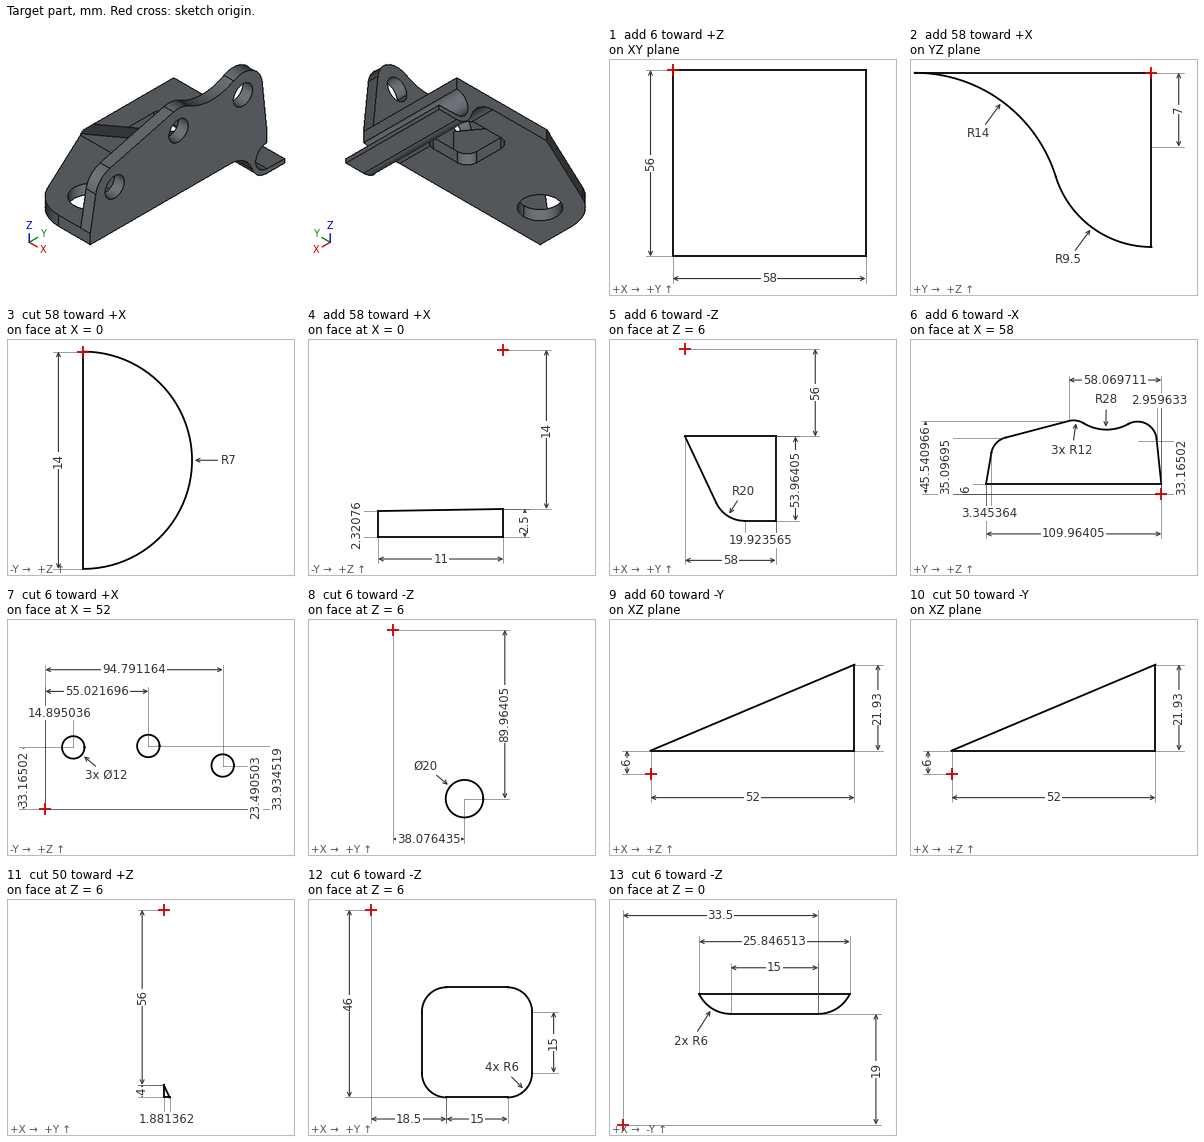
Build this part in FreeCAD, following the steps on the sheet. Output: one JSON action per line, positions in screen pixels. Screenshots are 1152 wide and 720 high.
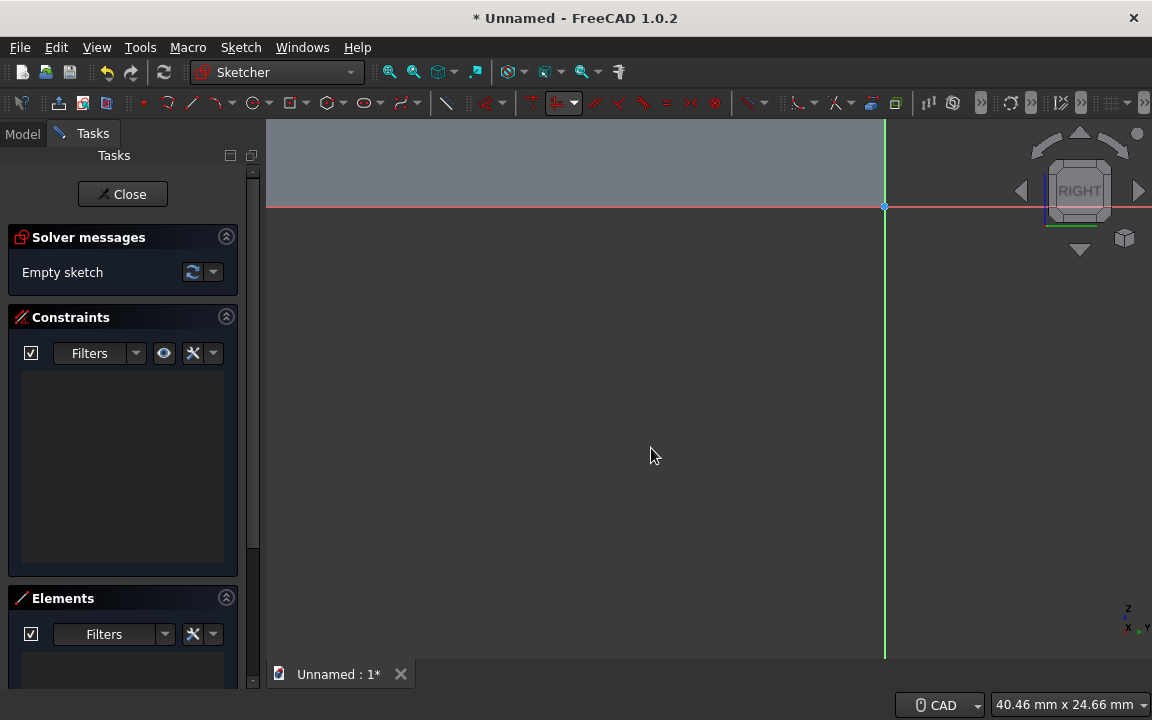
{"action": "left_click", "coordinate": [168, 104]}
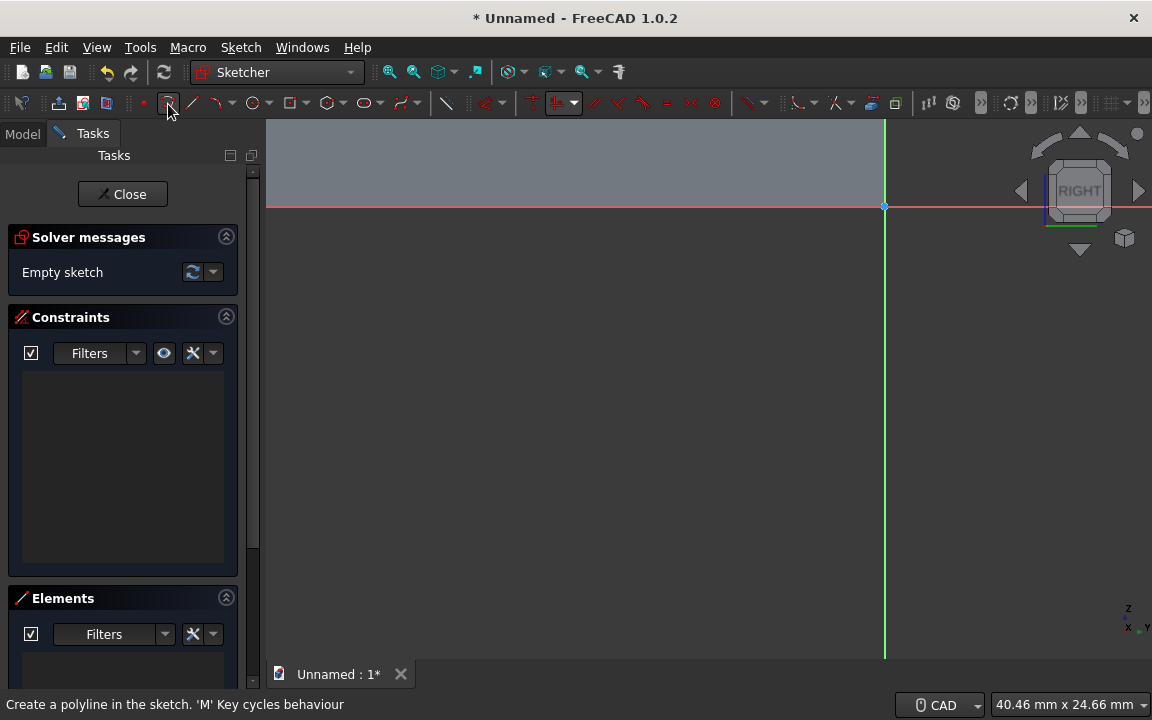
{"action": "left_click", "coordinate": [394, 207]}
{"action": "left_click", "coordinate": [885, 207]}
{"action": "left_click", "coordinate": [876, 568]}
{"action": "right_click", "coordinate": [876, 568]}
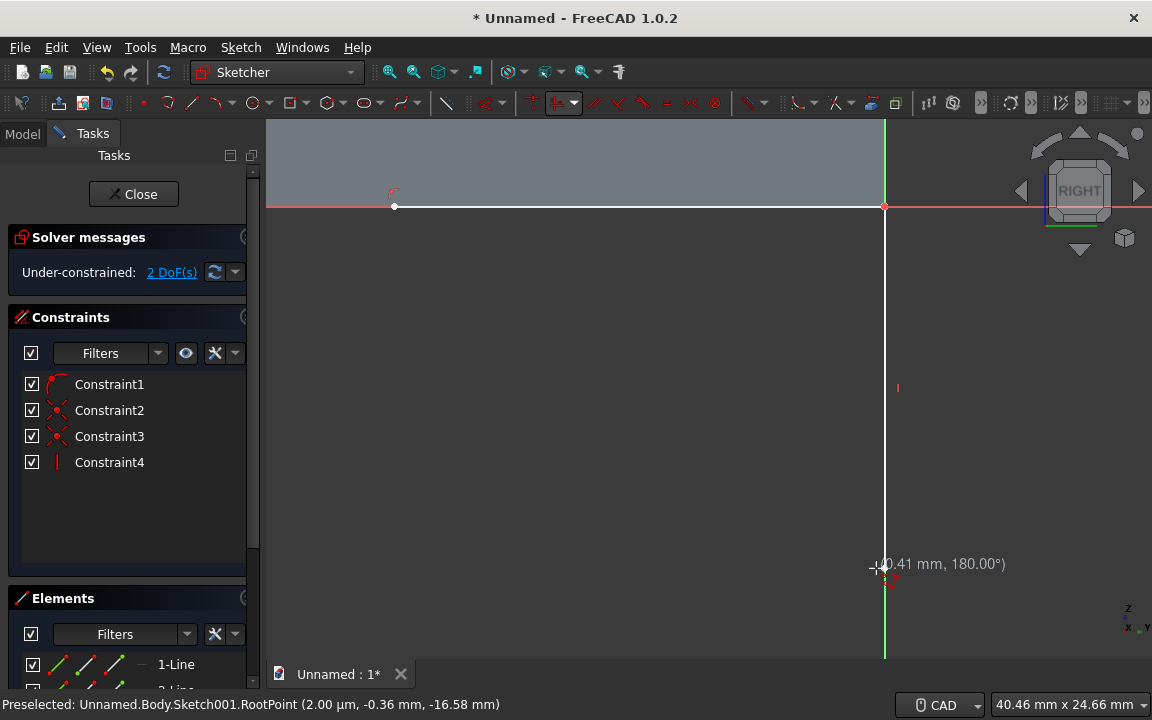
{"action": "left_click", "coordinate": [216, 104]}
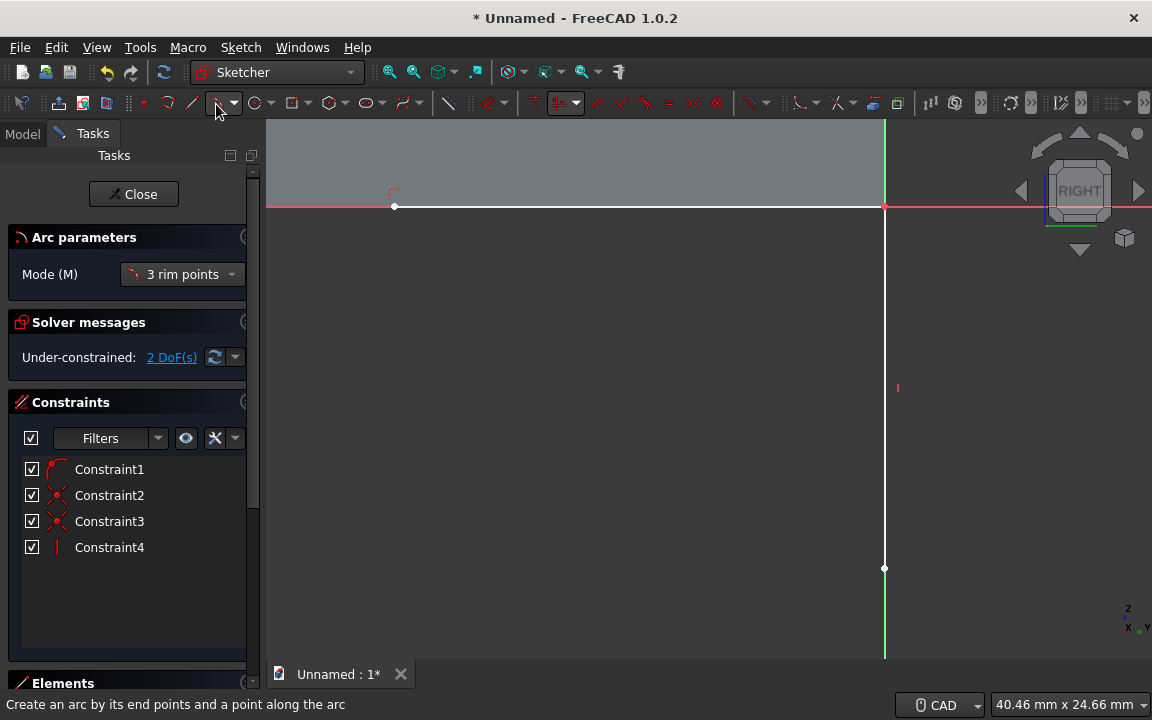
{"action": "left_click", "coordinate": [885, 569]}
{"action": "left_click", "coordinate": [686, 422]}
{"action": "left_click", "coordinate": [762, 528]}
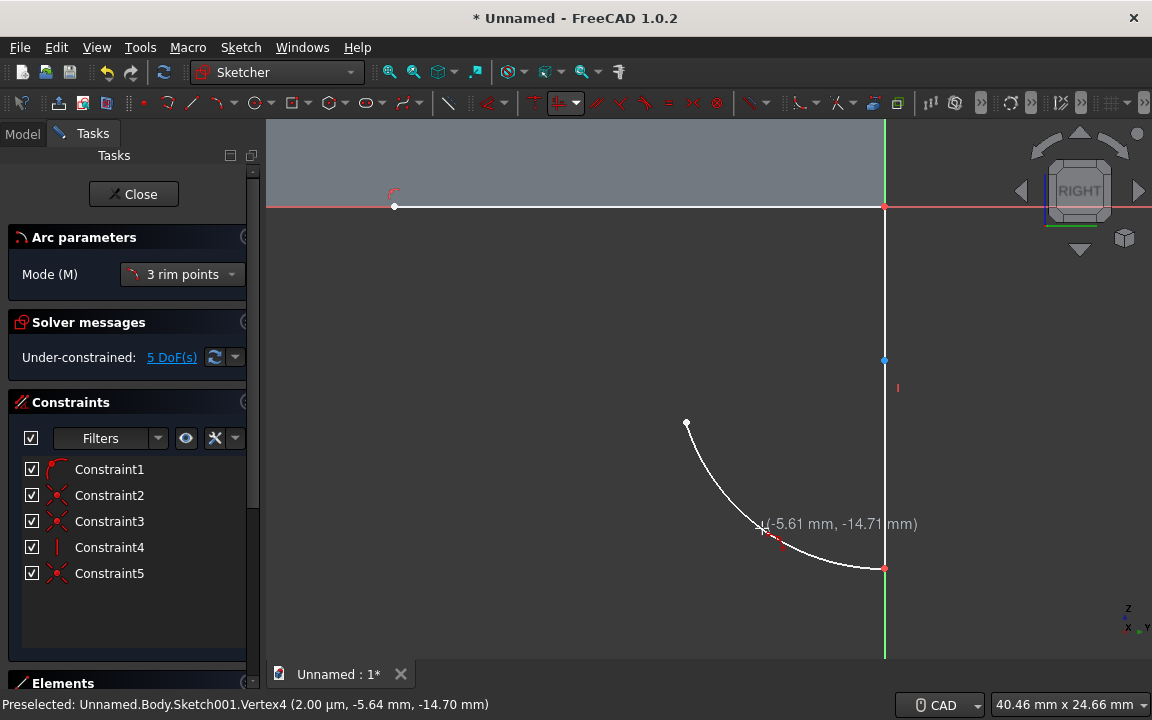
{"action": "left_click", "coordinate": [686, 423]}
{"action": "left_click", "coordinate": [394, 207]}
{"action": "left_click", "coordinate": [575, 266]}
{"action": "key", "text": "Escape"}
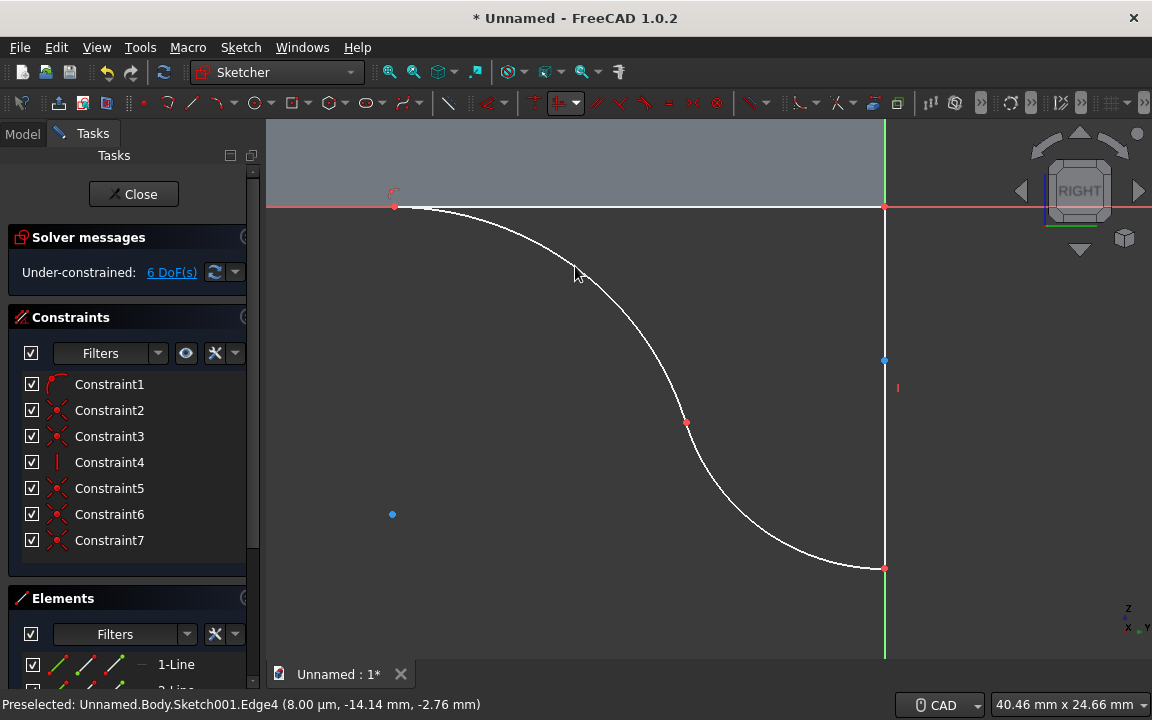
{"action": "left_click", "coordinate": [541, 207]}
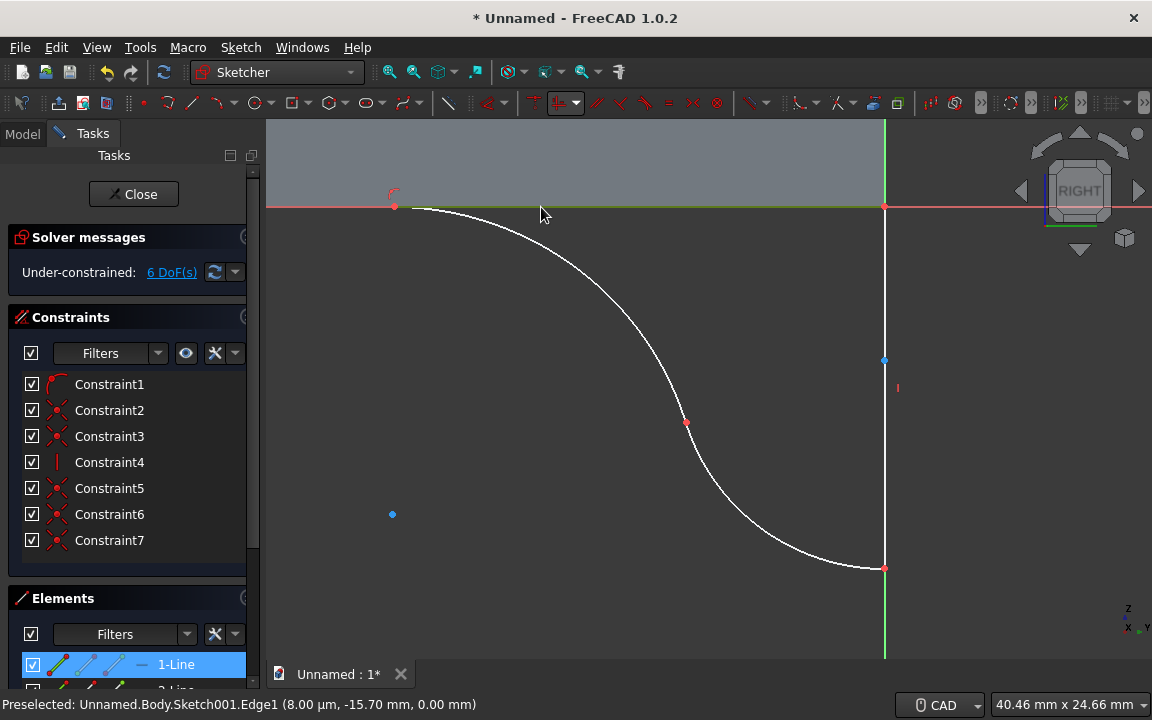
{"action": "left_click", "coordinate": [631, 321]}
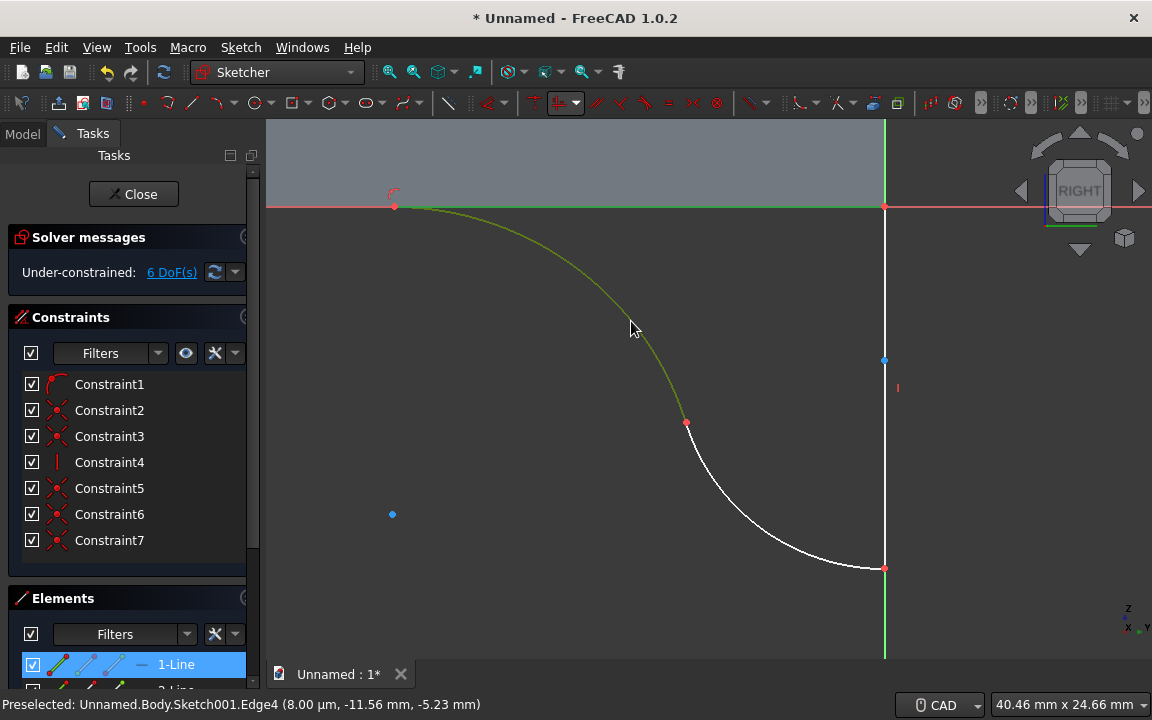
{"action": "left_click", "coordinate": [646, 104]}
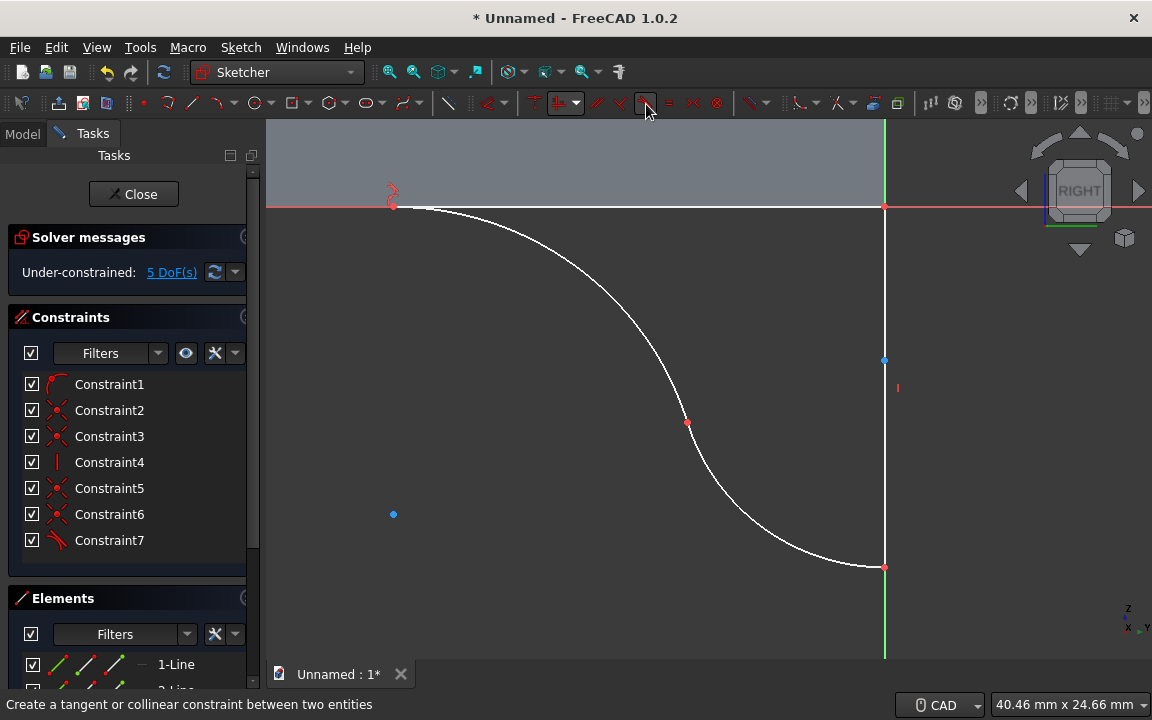
{"action": "left_click", "coordinate": [725, 492]}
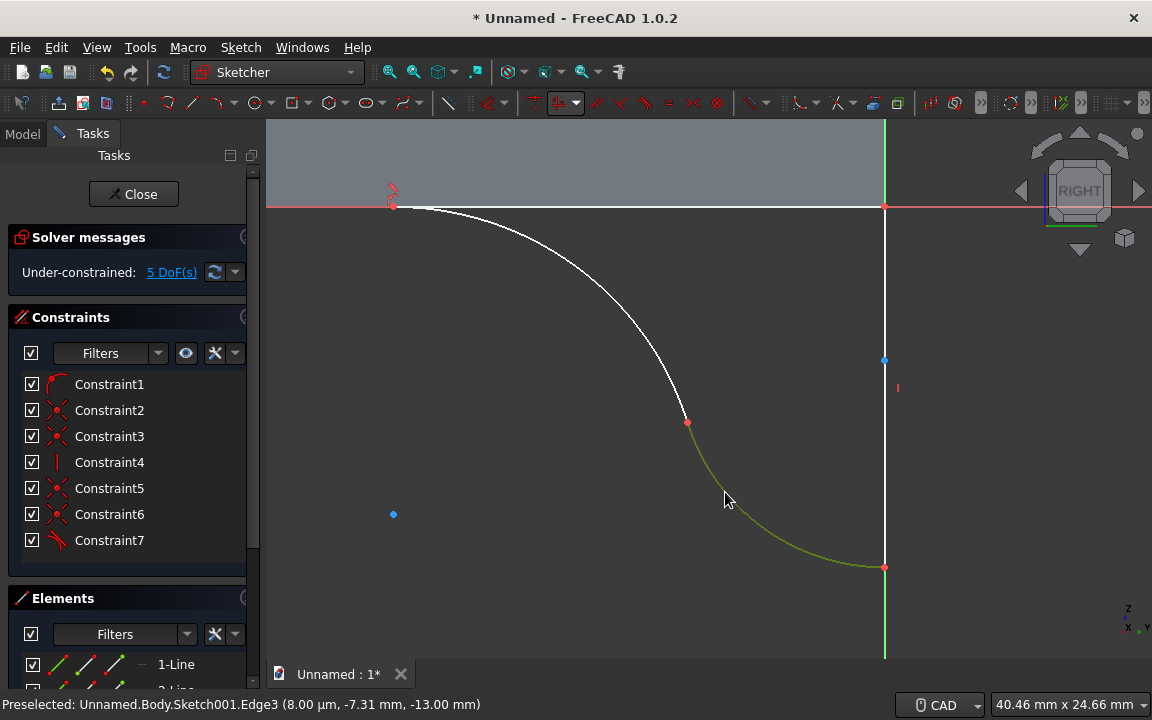
{"action": "left_click", "coordinate": [633, 320]}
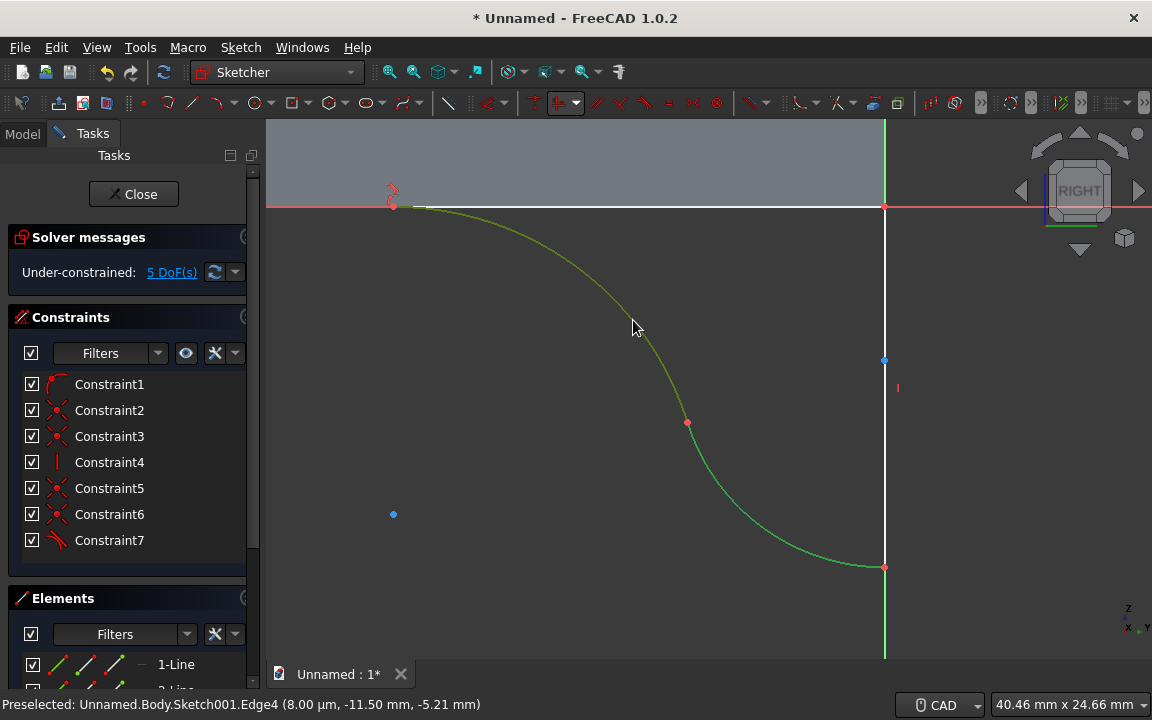
{"action": "left_click", "coordinate": [646, 104]}